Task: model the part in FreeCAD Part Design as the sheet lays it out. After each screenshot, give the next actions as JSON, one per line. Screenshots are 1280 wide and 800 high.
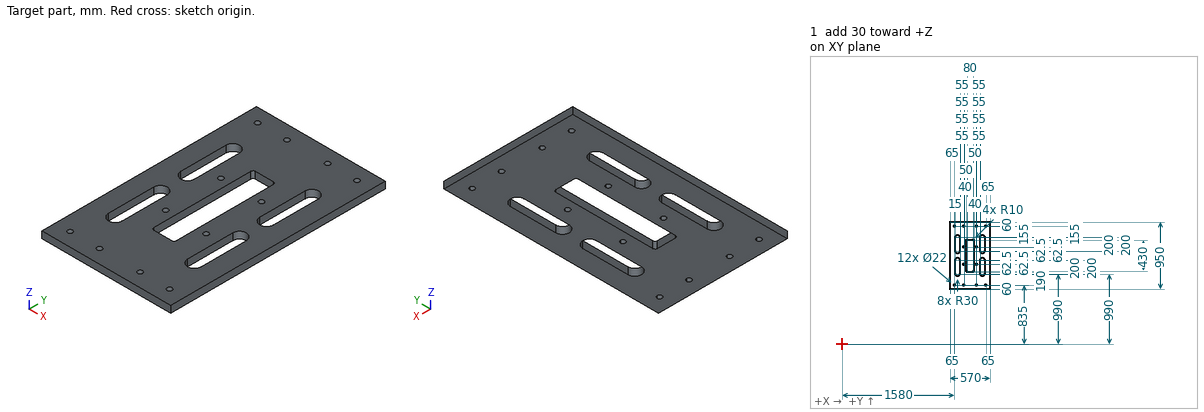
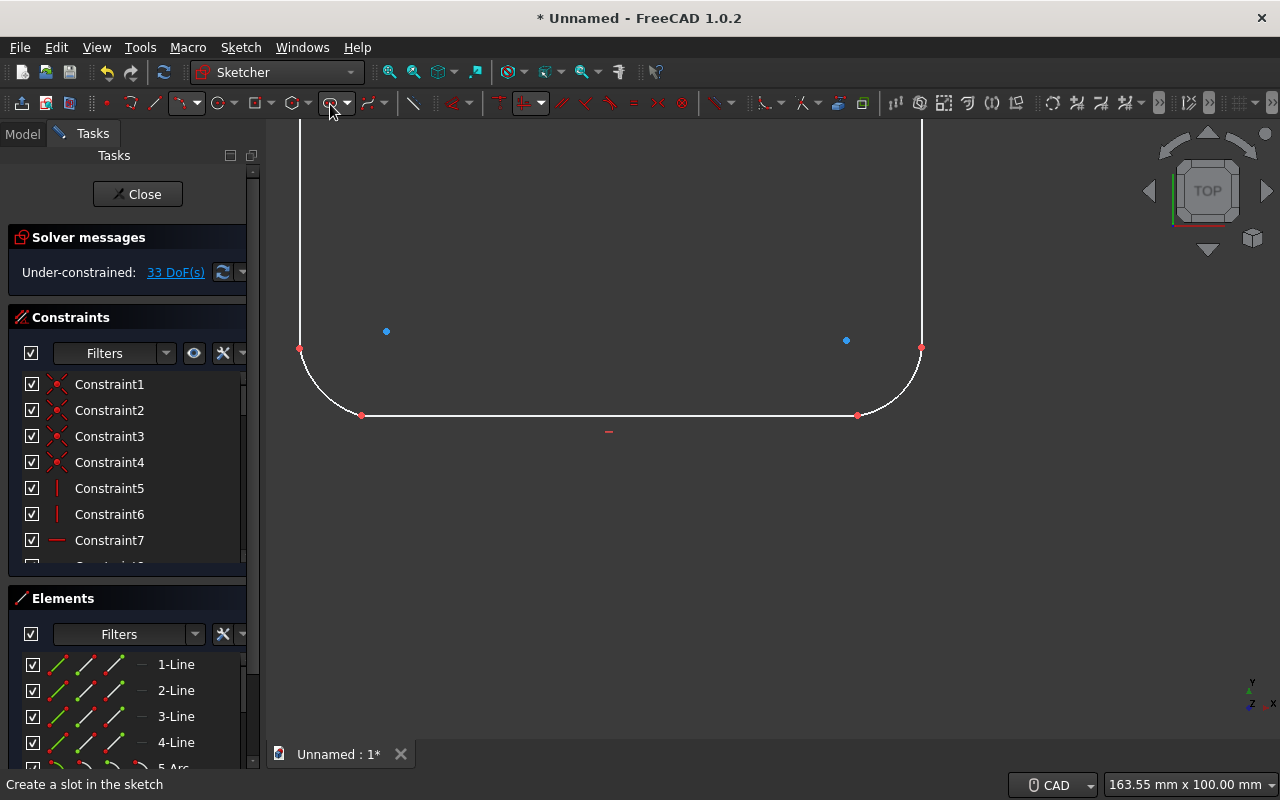
{"action": "scroll", "coordinate": [908, 387], "scroll_direction": "down", "scroll_amount": 16}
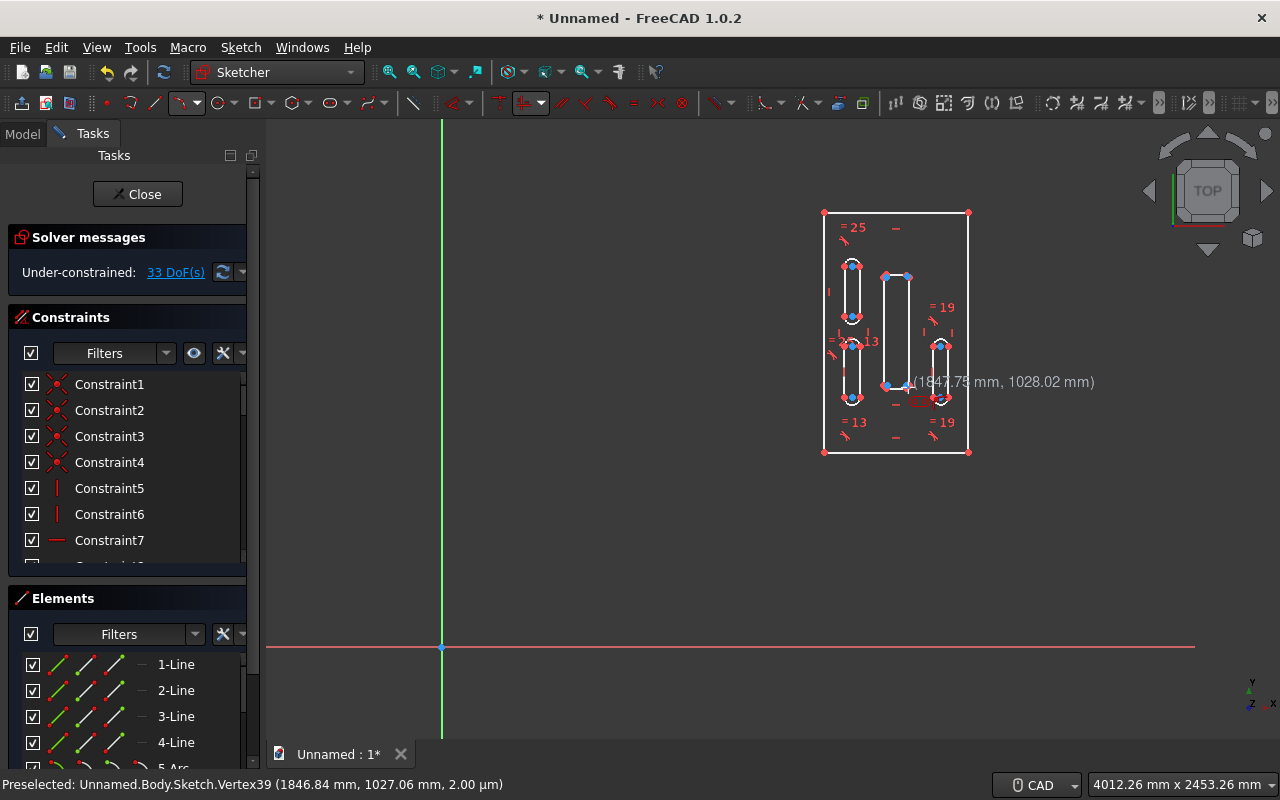
{"action": "scroll", "coordinate": [941, 316], "scroll_direction": "up", "scroll_amount": 6}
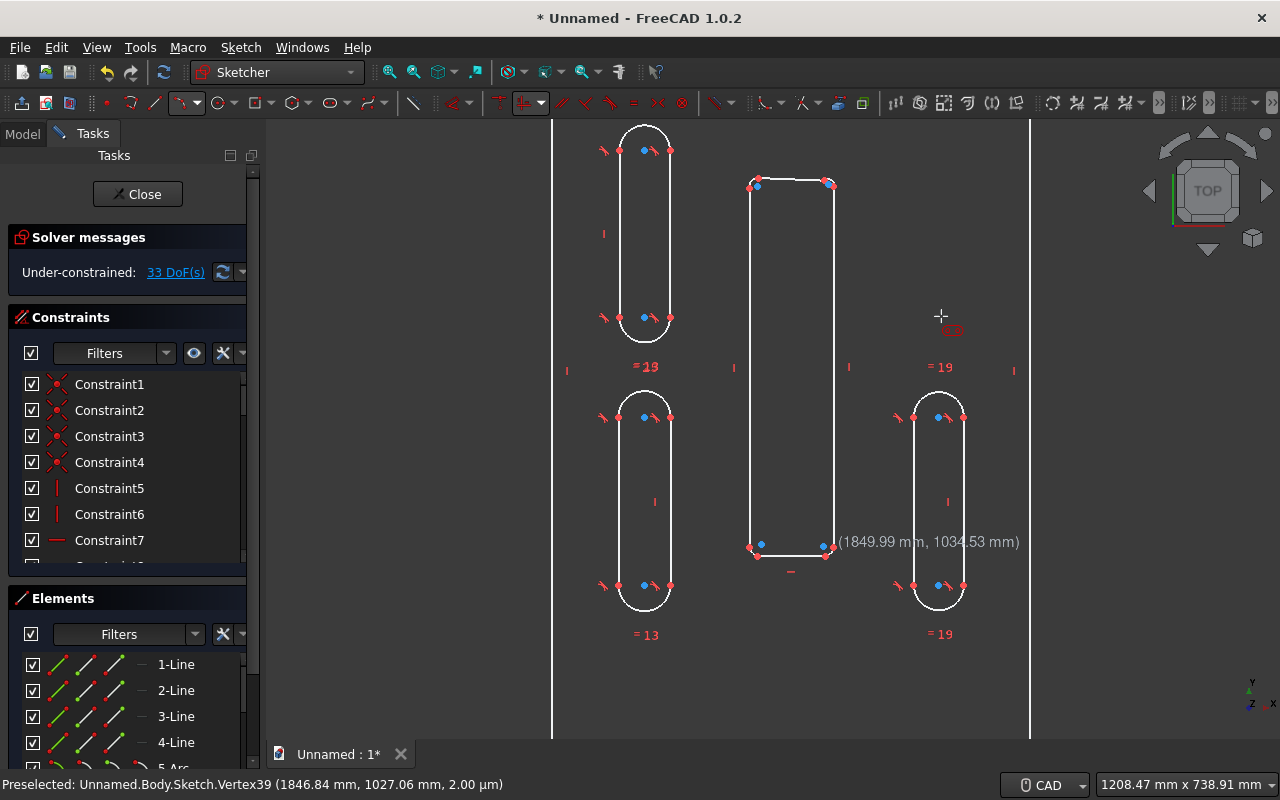
{"action": "left_click", "coordinate": [939, 316]}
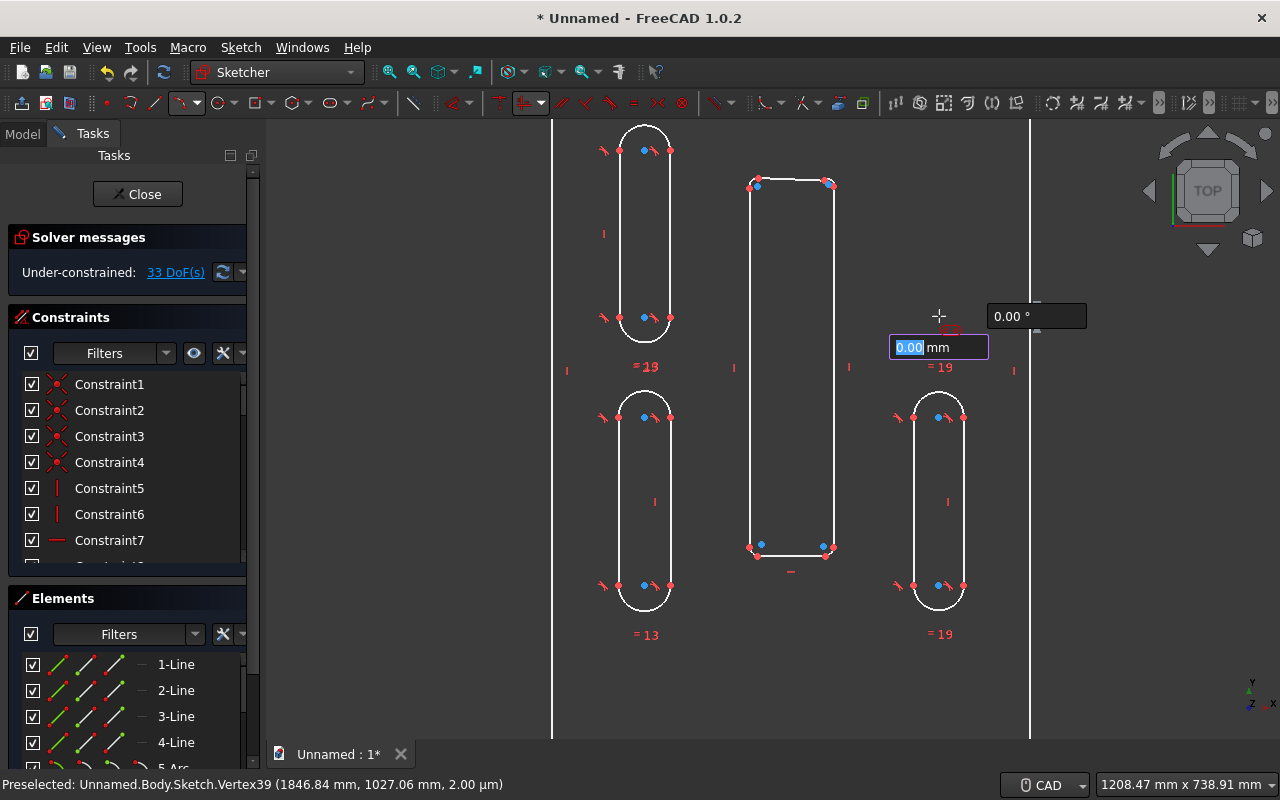
{"action": "left_click", "coordinate": [939, 148]}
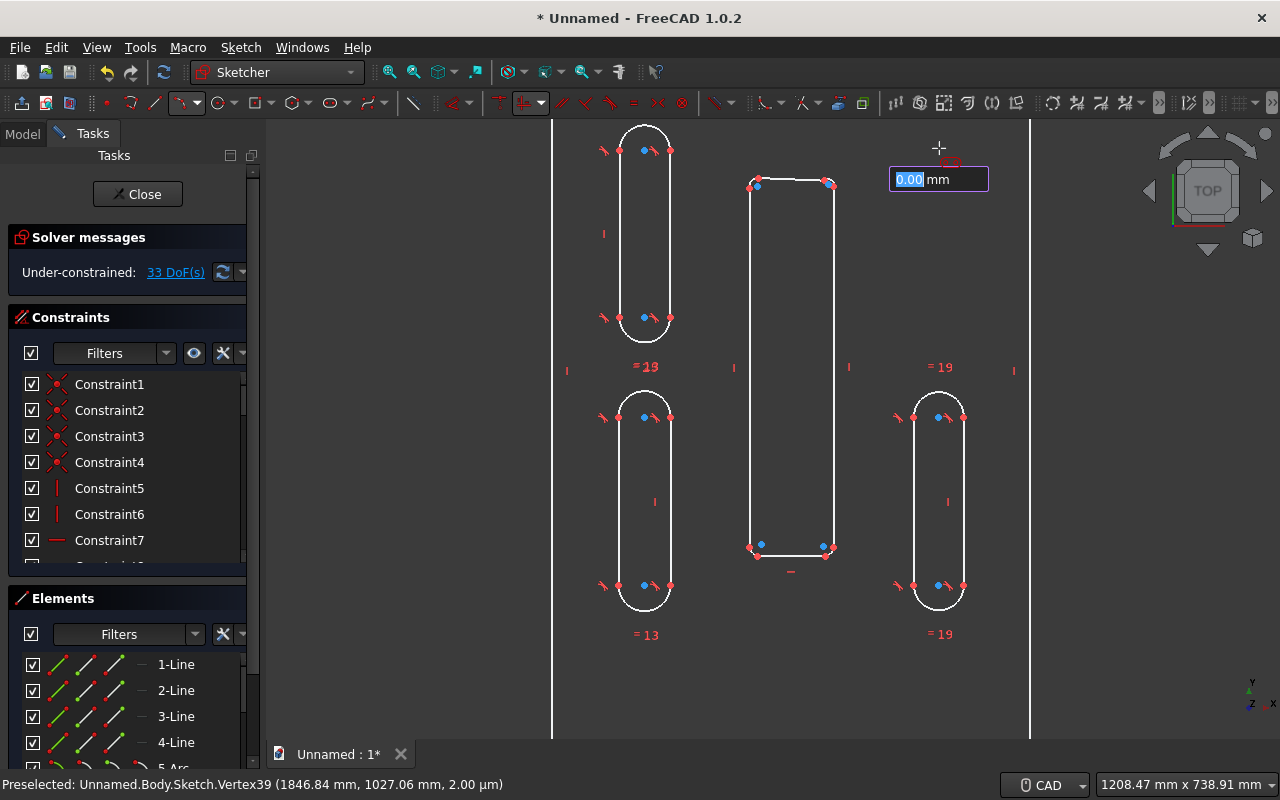
{"action": "left_click", "coordinate": [964, 232]}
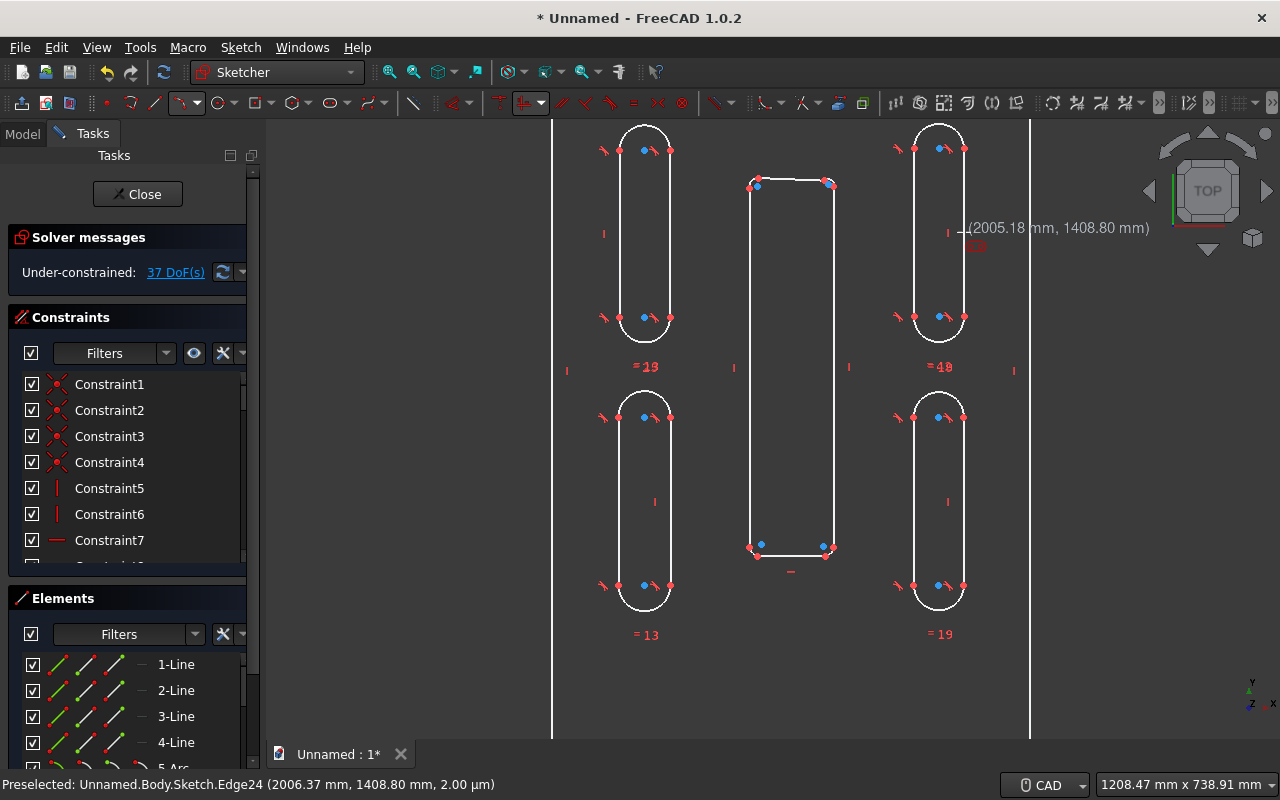
{"action": "left_click", "coordinate": [218, 104]}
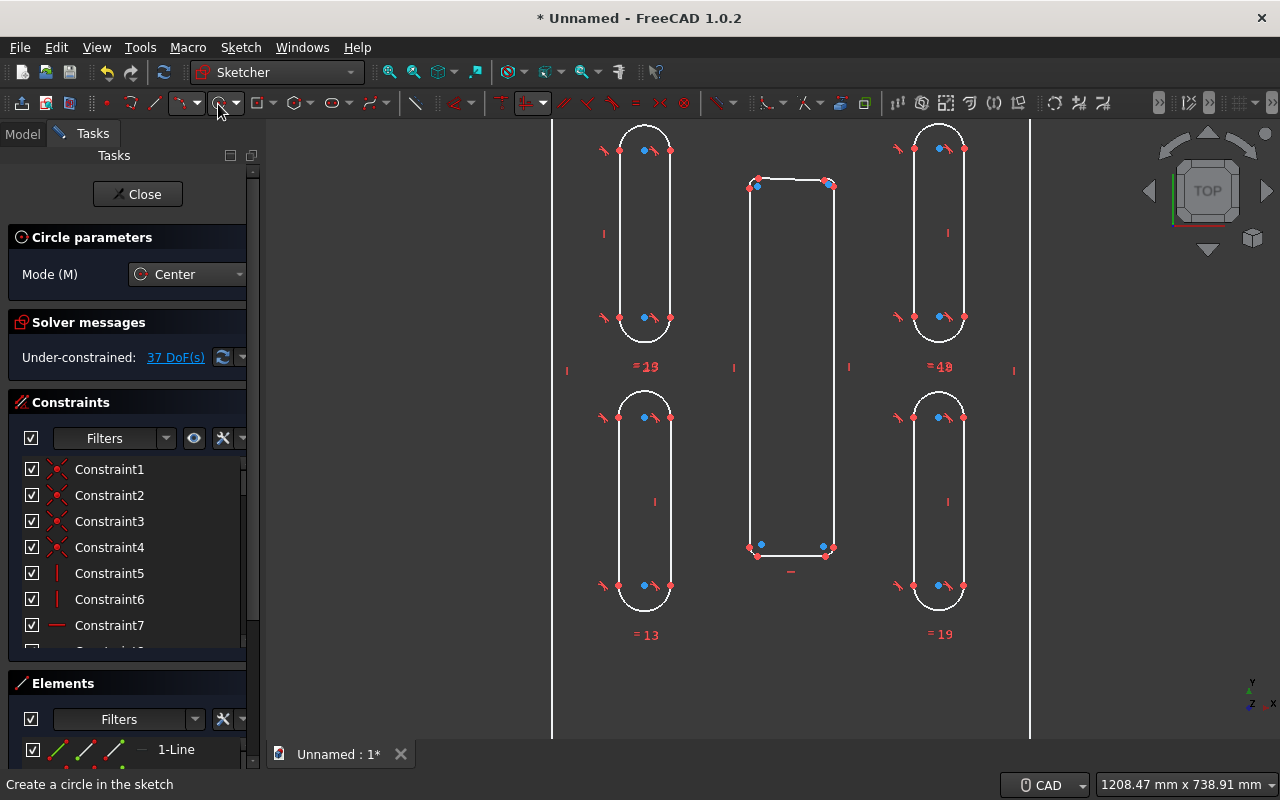
{"action": "scroll", "coordinate": [941, 316], "scroll_direction": "down", "scroll_amount": 6}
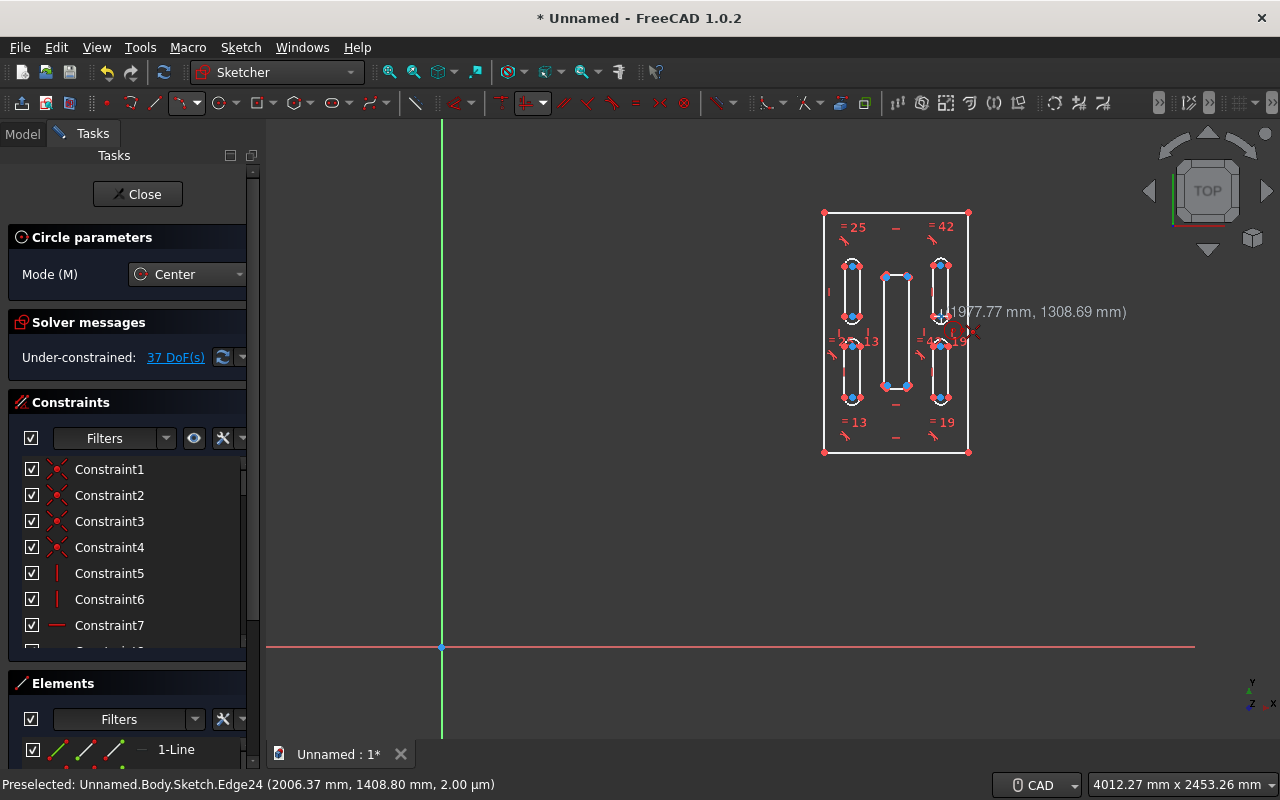
{"action": "scroll", "coordinate": [841, 436], "scroll_direction": "up", "scroll_amount": 11}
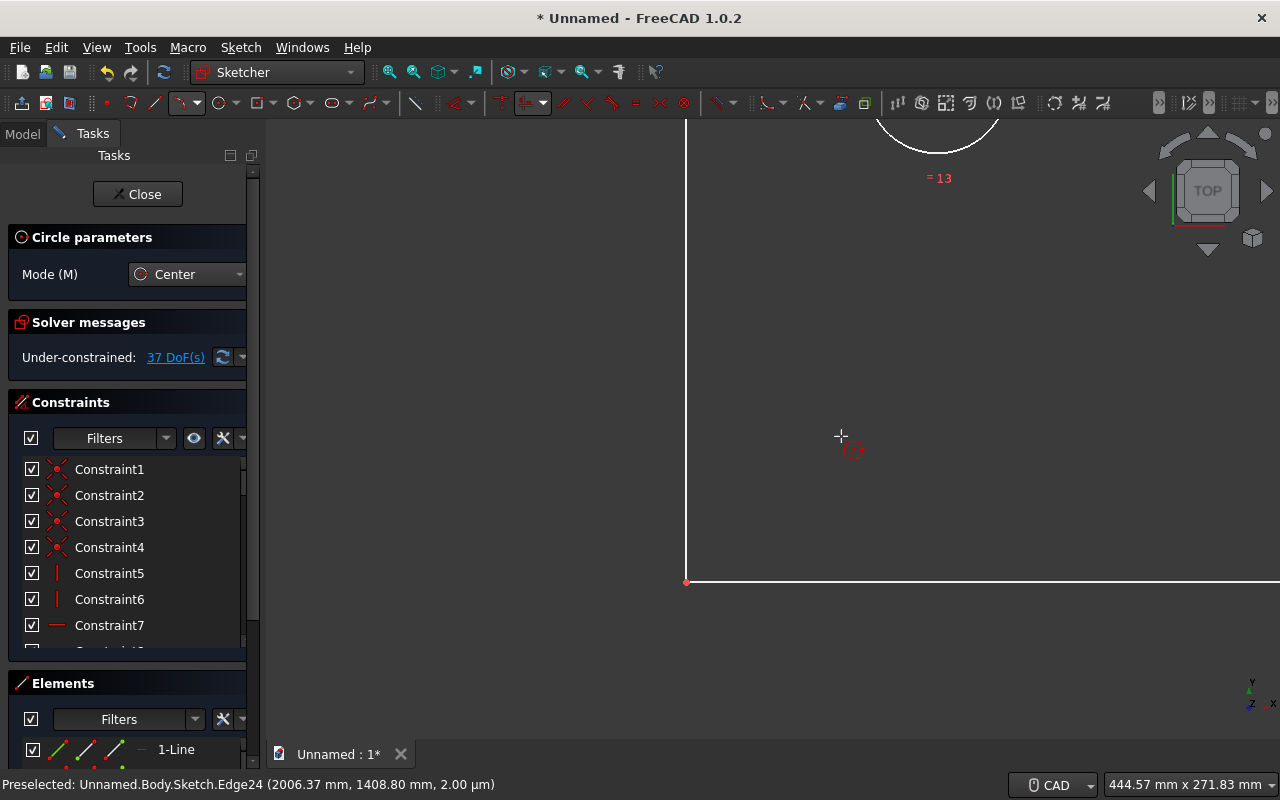
{"action": "scroll", "coordinate": [841, 436], "scroll_direction": "down", "scroll_amount": 11}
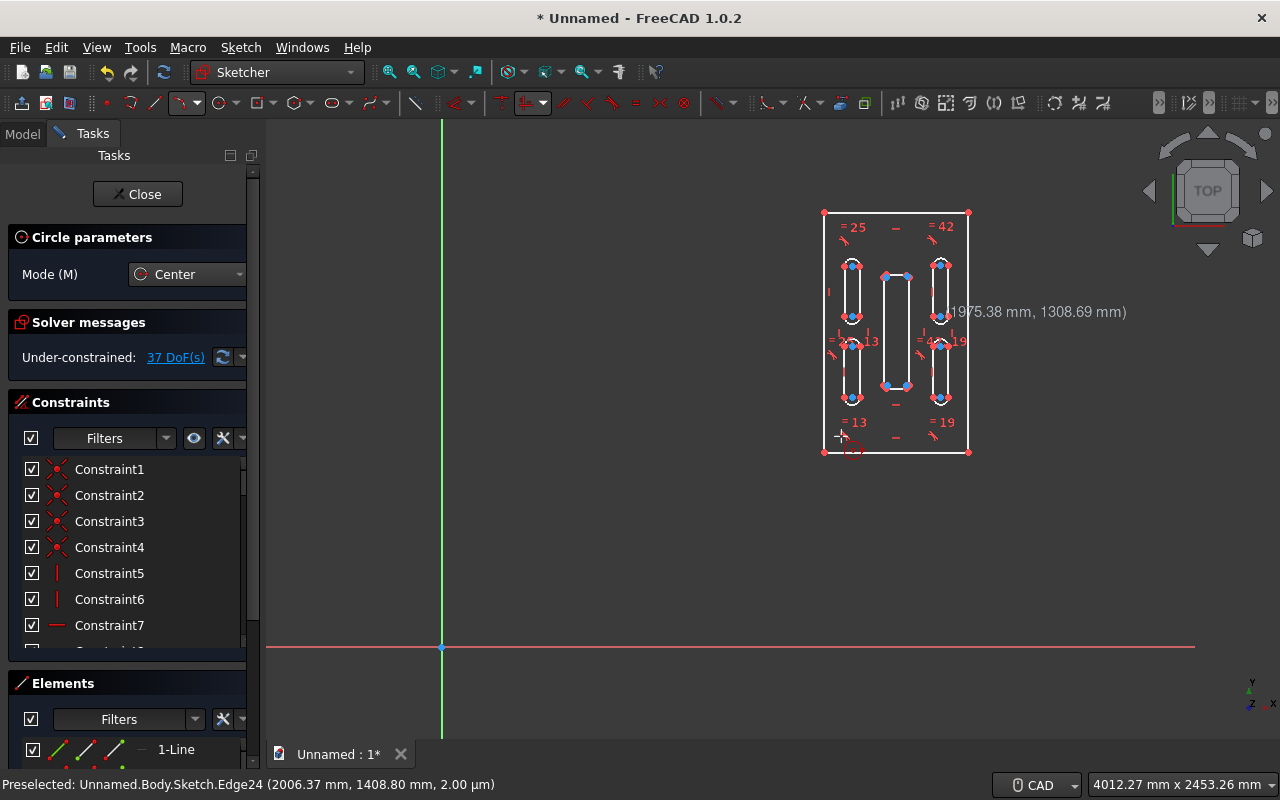
{"action": "left_click", "coordinate": [841, 436]}